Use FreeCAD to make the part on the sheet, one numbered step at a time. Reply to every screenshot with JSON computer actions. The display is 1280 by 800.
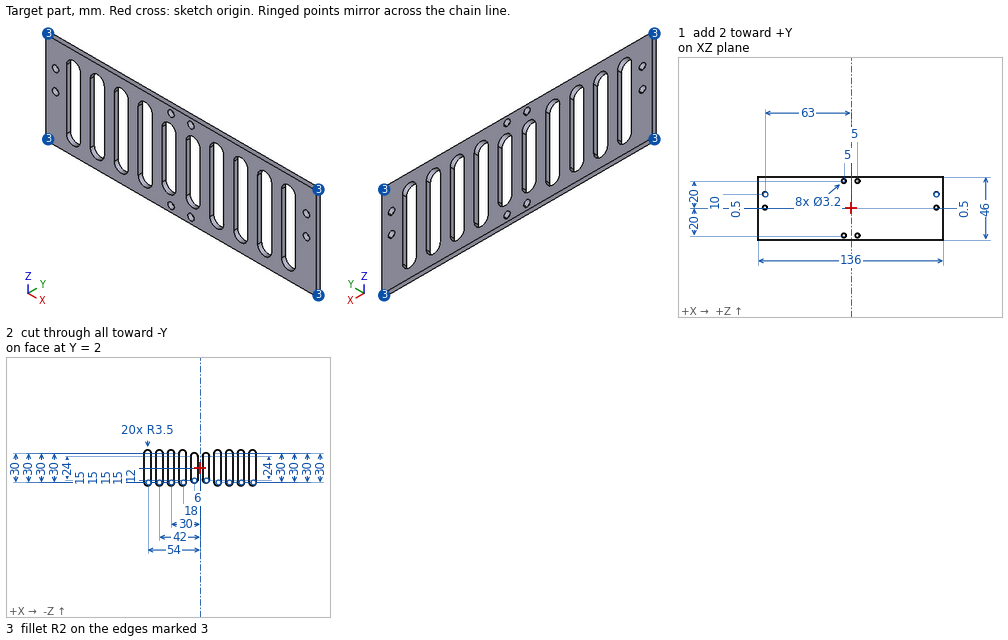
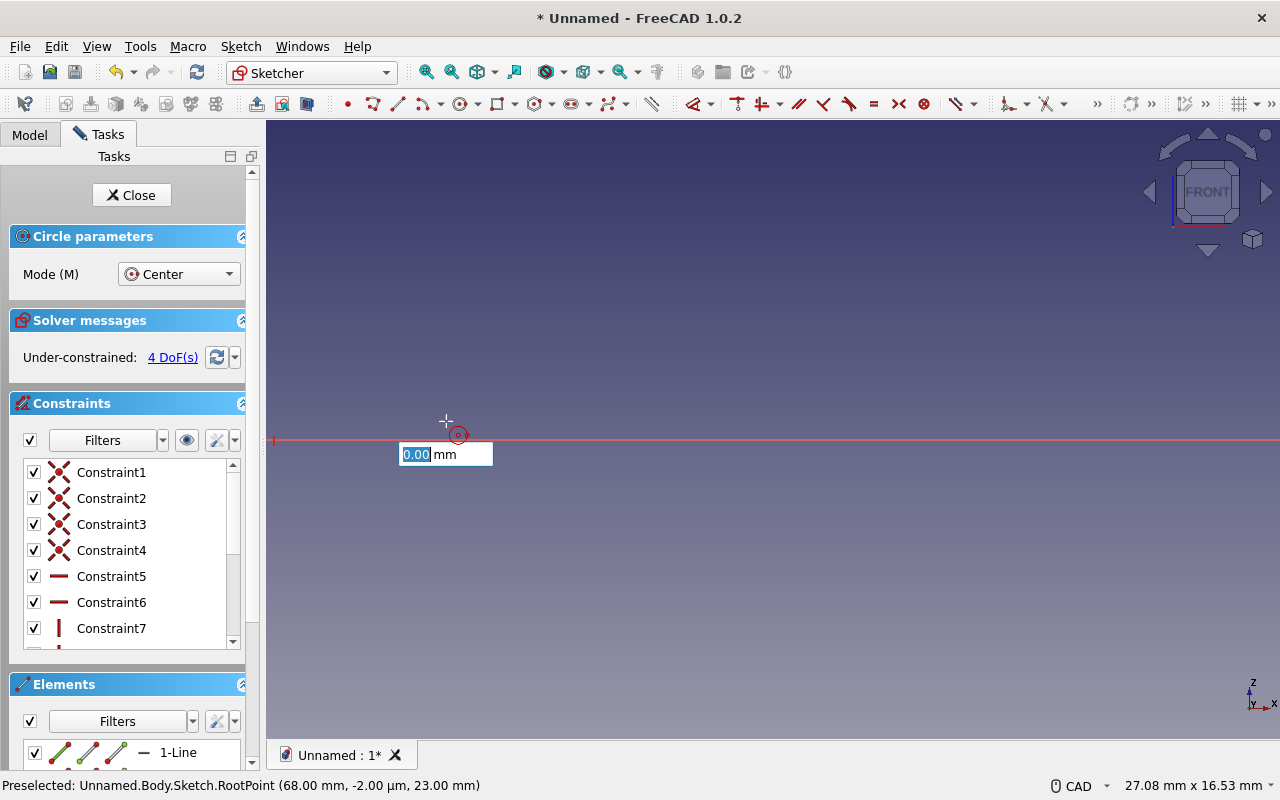
{"action": "scroll", "coordinate": [443, 428], "scroll_direction": "down", "scroll_amount": 11}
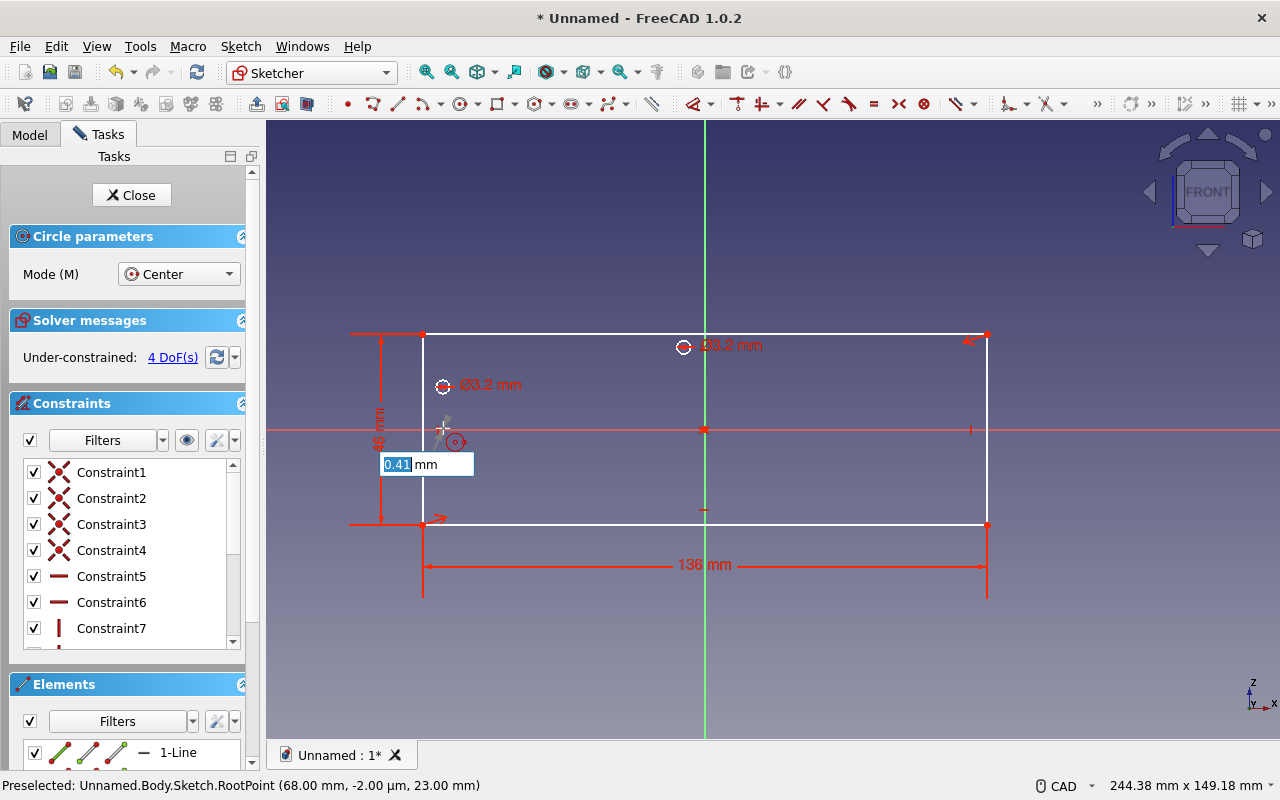
{"action": "scroll", "coordinate": [448, 423], "scroll_direction": "up", "scroll_amount": 5}
{"action": "mouse_move", "coordinate": [448, 422]}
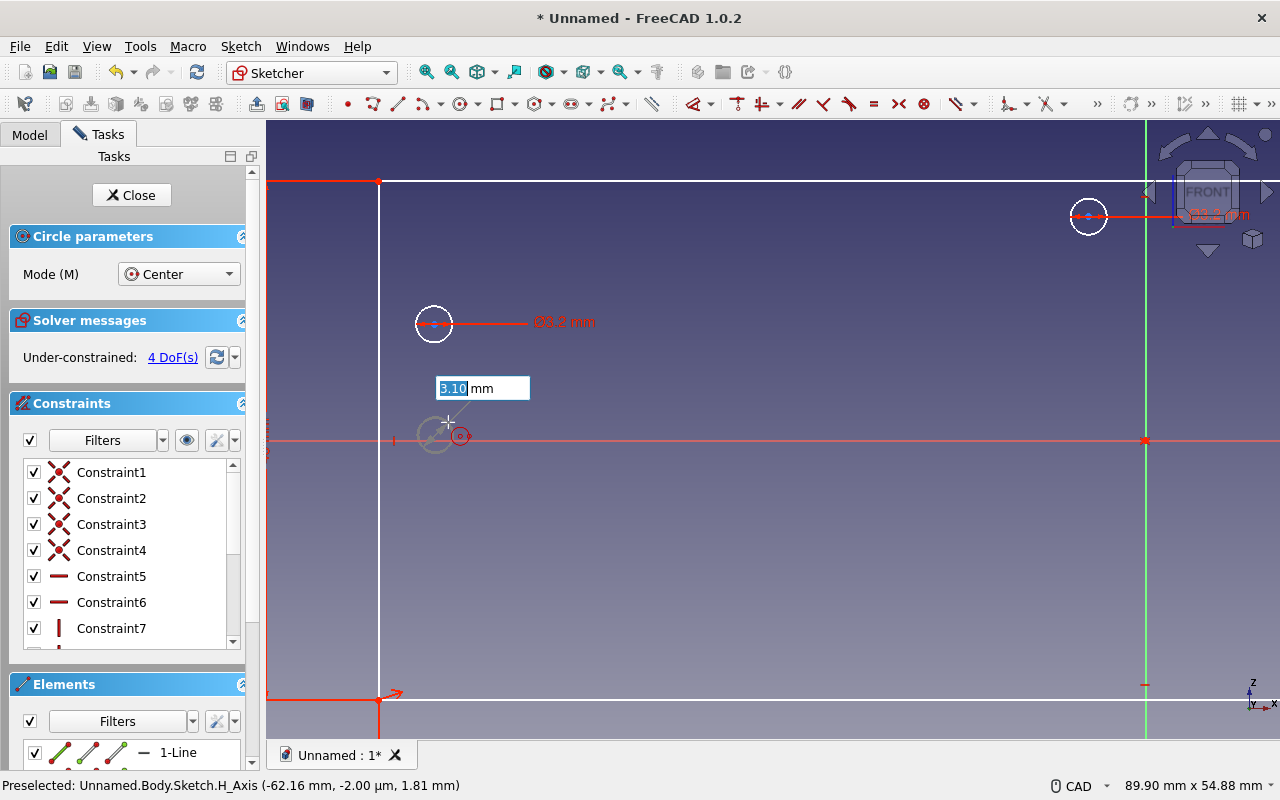
{"action": "type", "text": "3.2"}
{"action": "key", "text": "Return"}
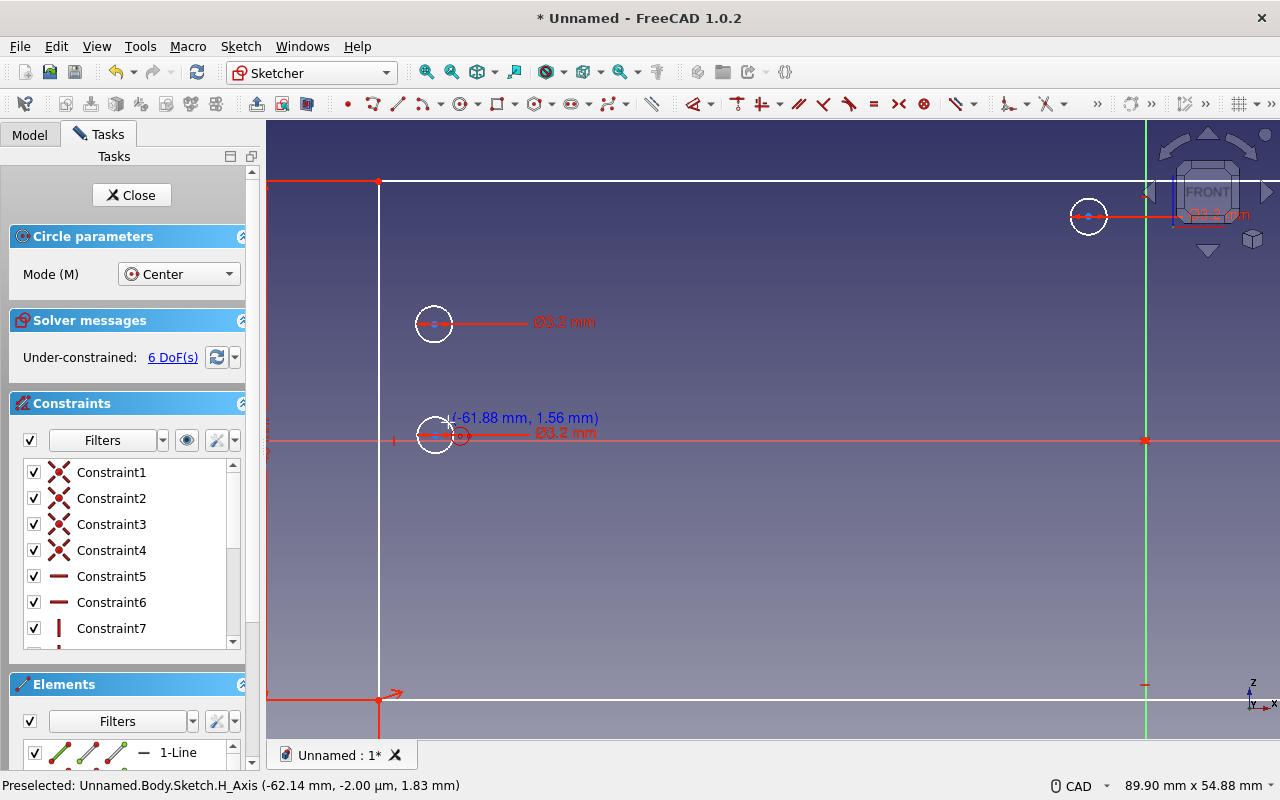
{"action": "scroll", "coordinate": [448, 423], "scroll_direction": "down", "scroll_amount": 5}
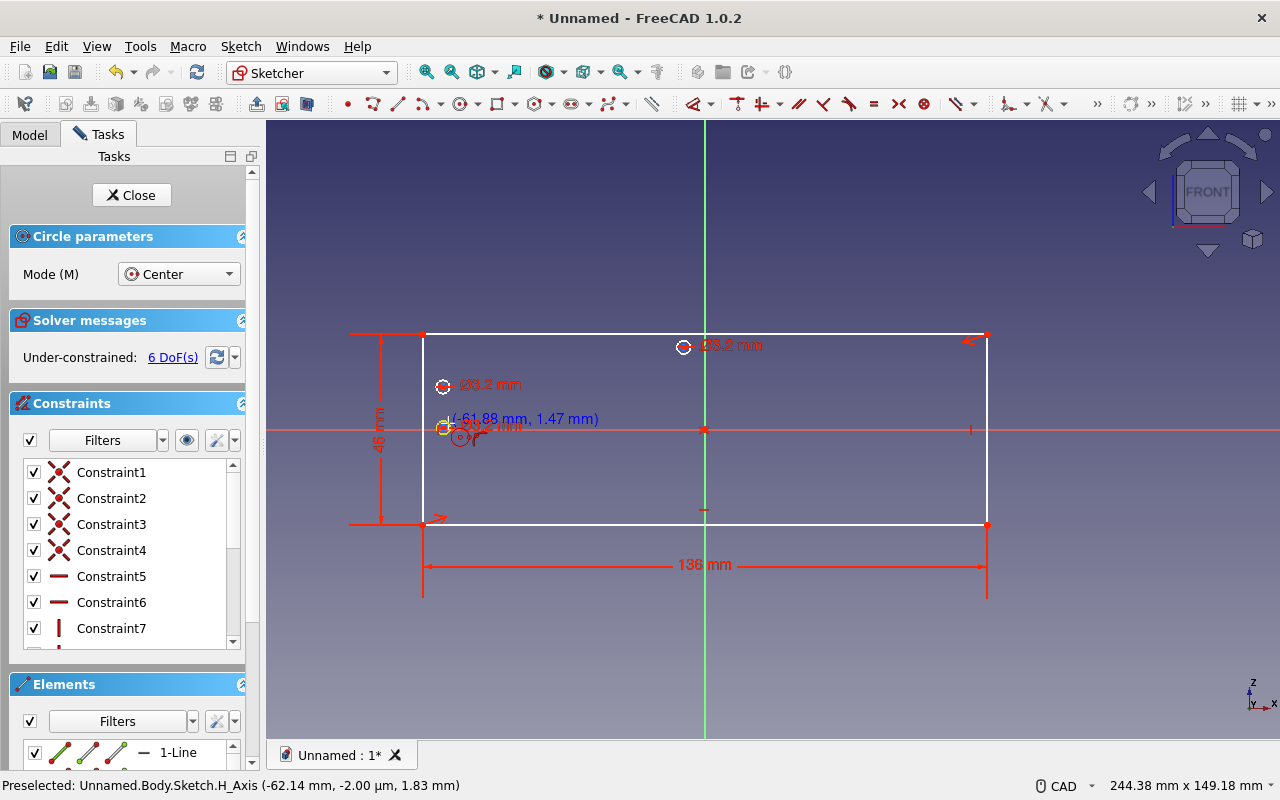
{"action": "scroll", "coordinate": [726, 347], "scroll_direction": "up", "scroll_amount": 7}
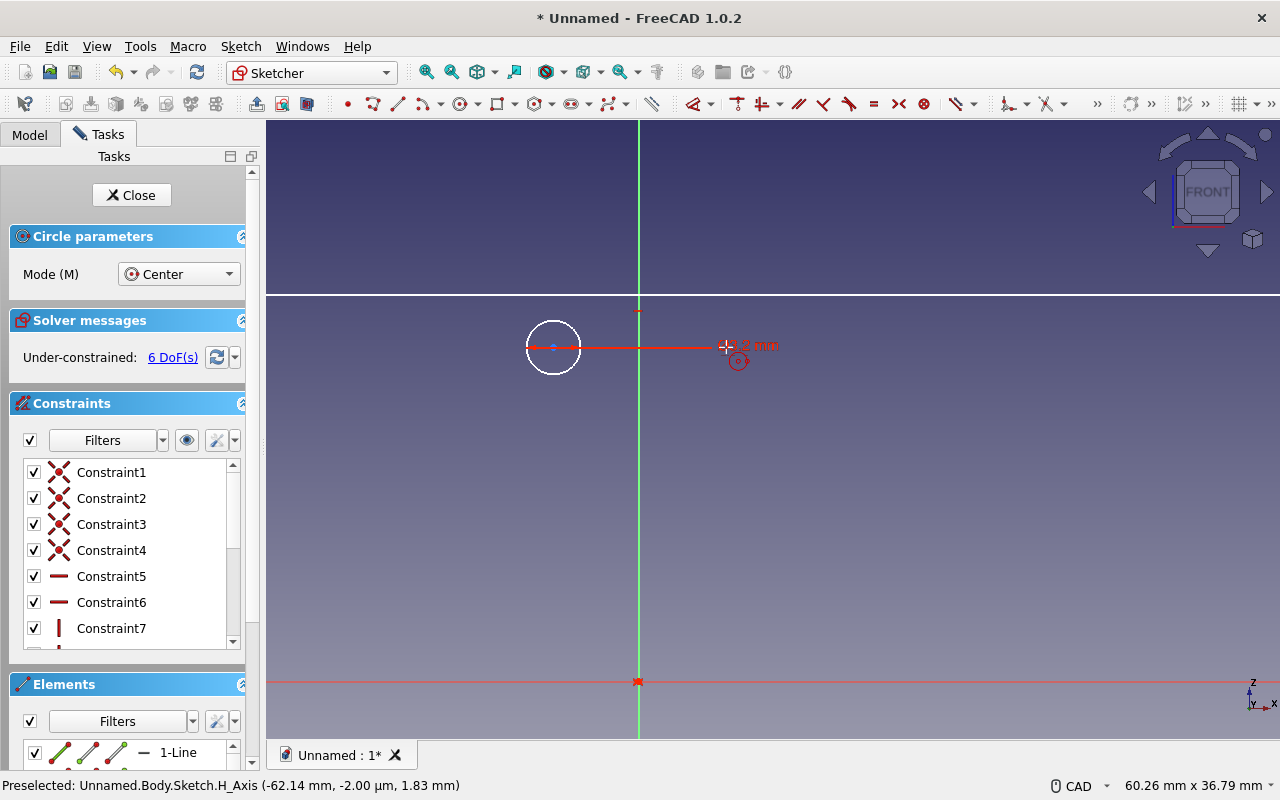
{"action": "scroll", "coordinate": [726, 347], "scroll_direction": "down", "scroll_amount": 7}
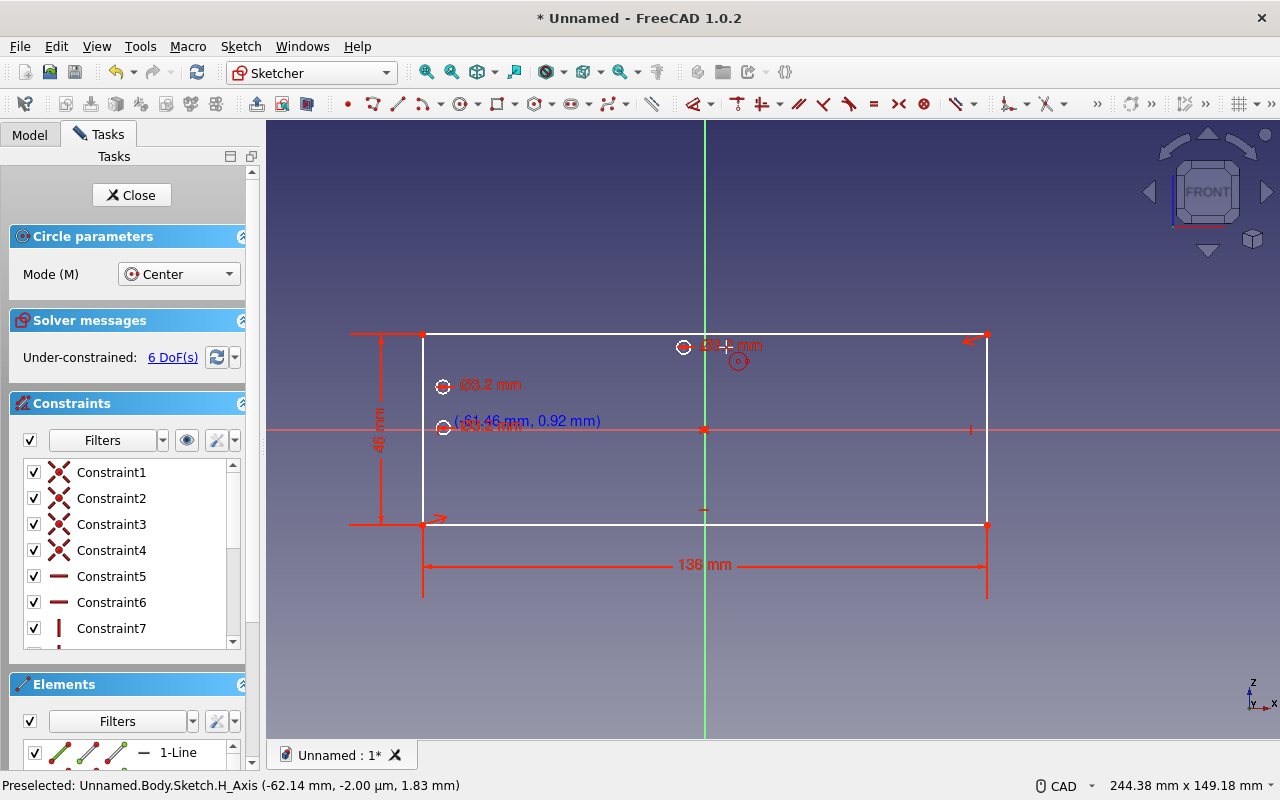
{"action": "scroll", "coordinate": [726, 347], "scroll_direction": "up", "scroll_amount": 2}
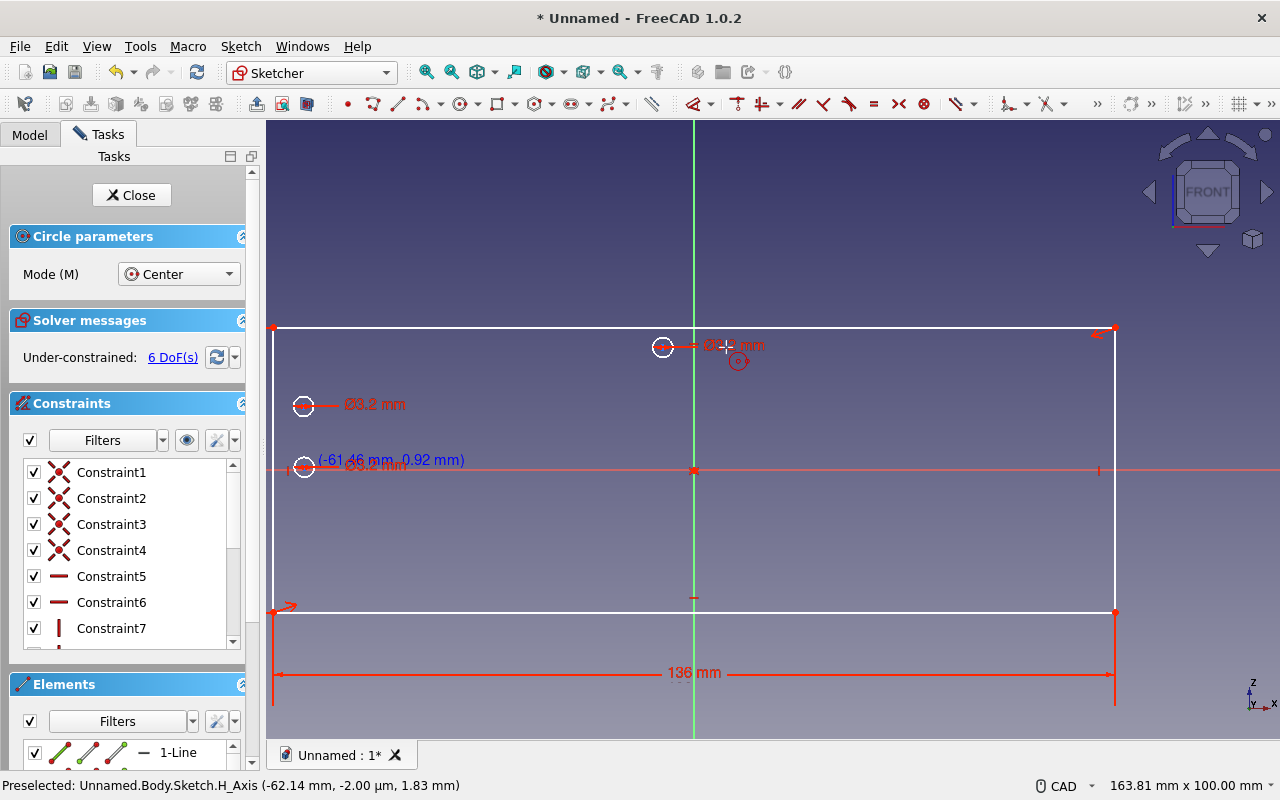
{"action": "left_click", "coordinate": [725, 347]}
{"action": "mouse_move", "coordinate": [732, 354]}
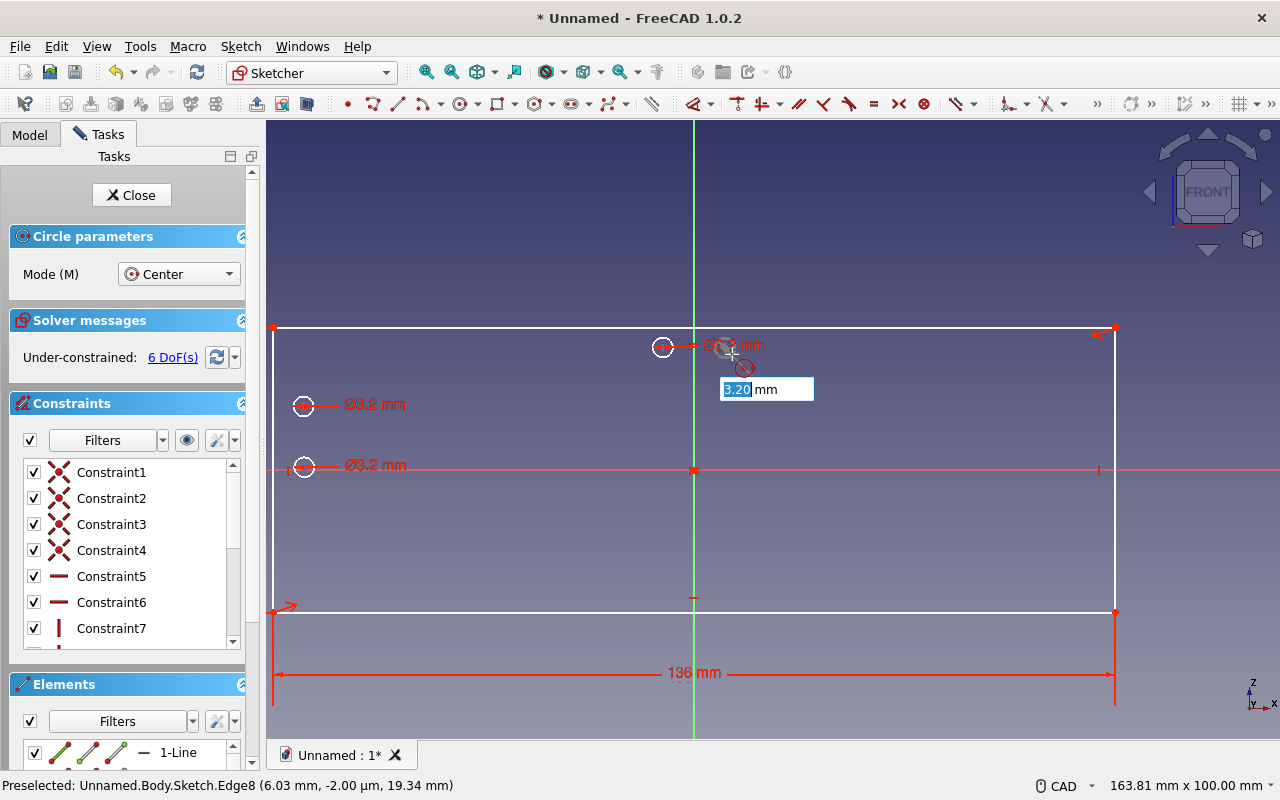
{"action": "type", "text": "3.2"}
{"action": "key", "text": "Return"}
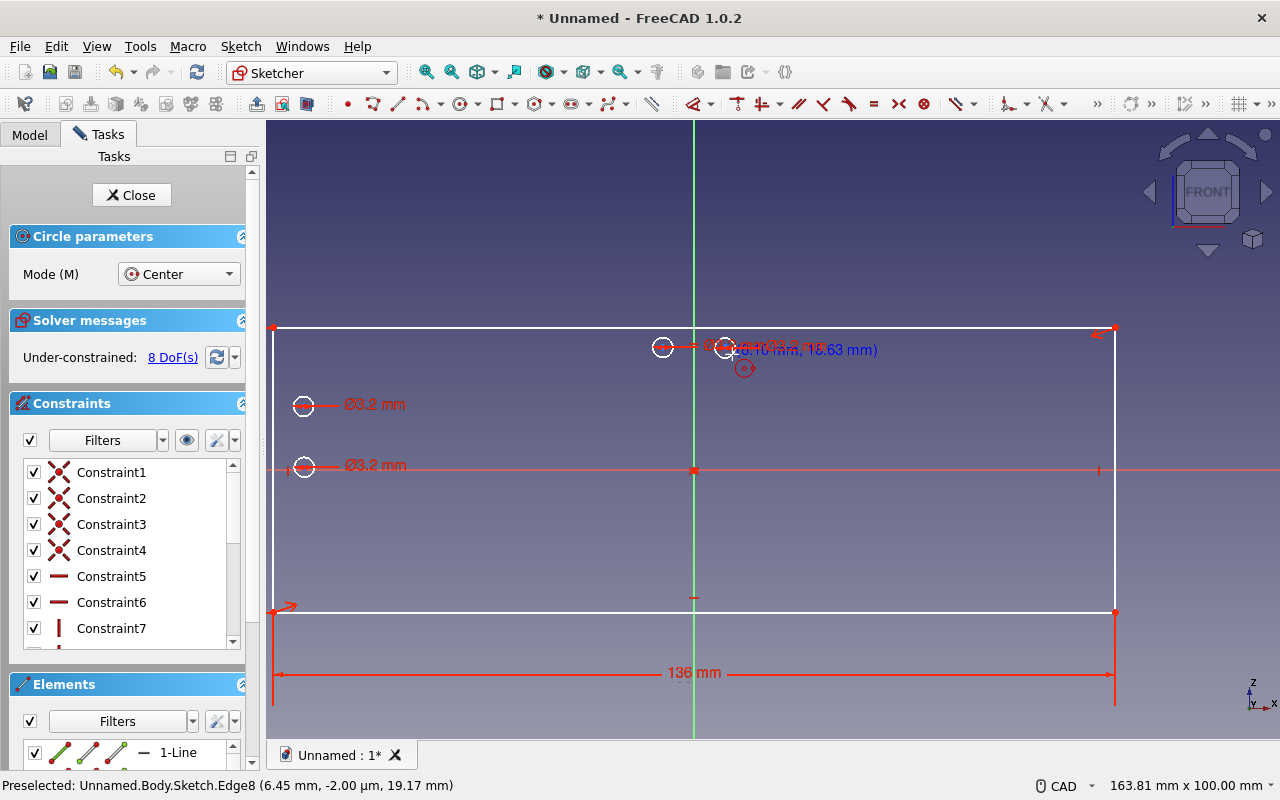
{"action": "scroll", "coordinate": [1084, 405], "scroll_direction": "up", "scroll_amount": 5}